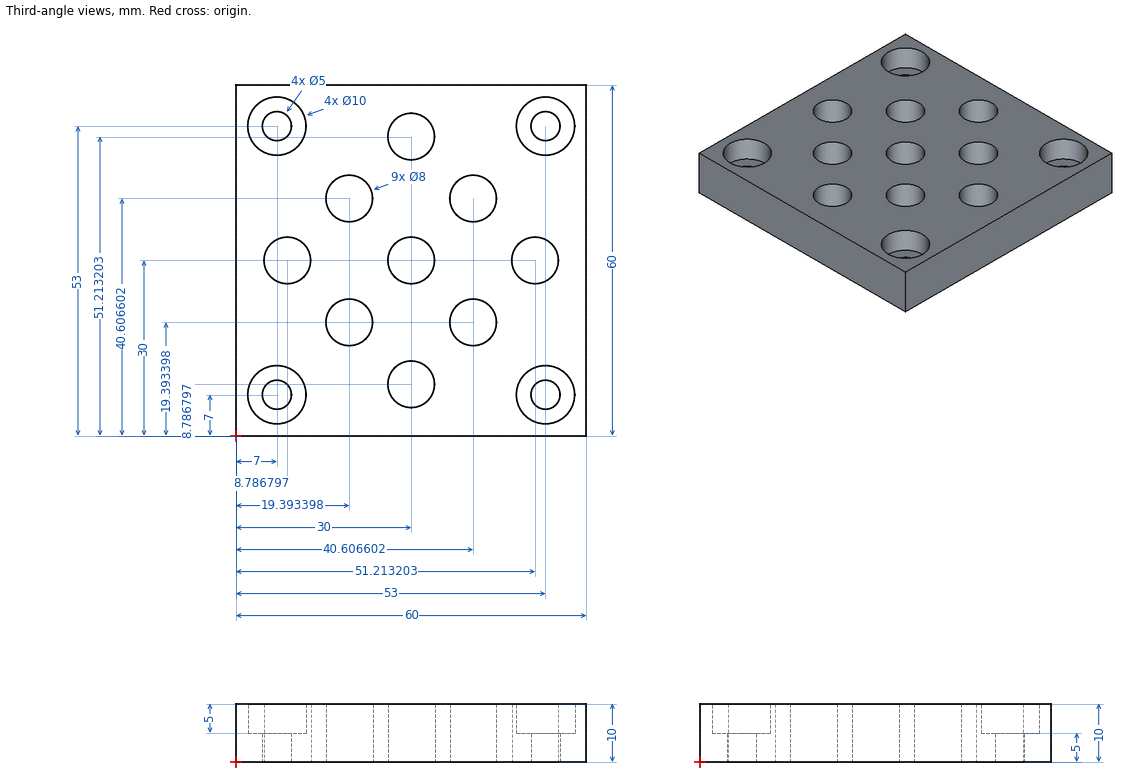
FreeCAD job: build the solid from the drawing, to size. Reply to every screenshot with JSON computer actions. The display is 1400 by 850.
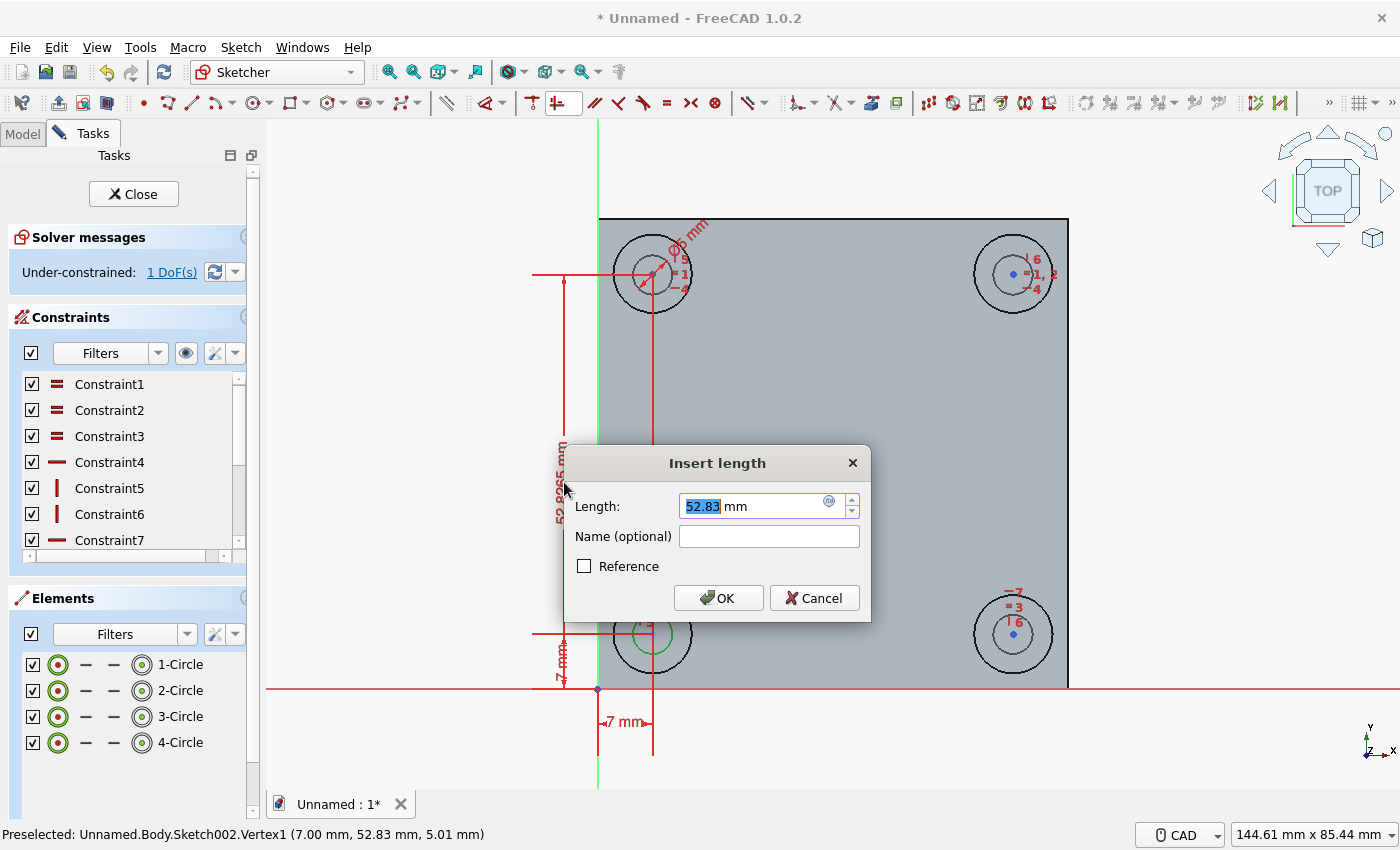
{"action": "type", "text": "53"}
{"action": "key", "text": "Return"}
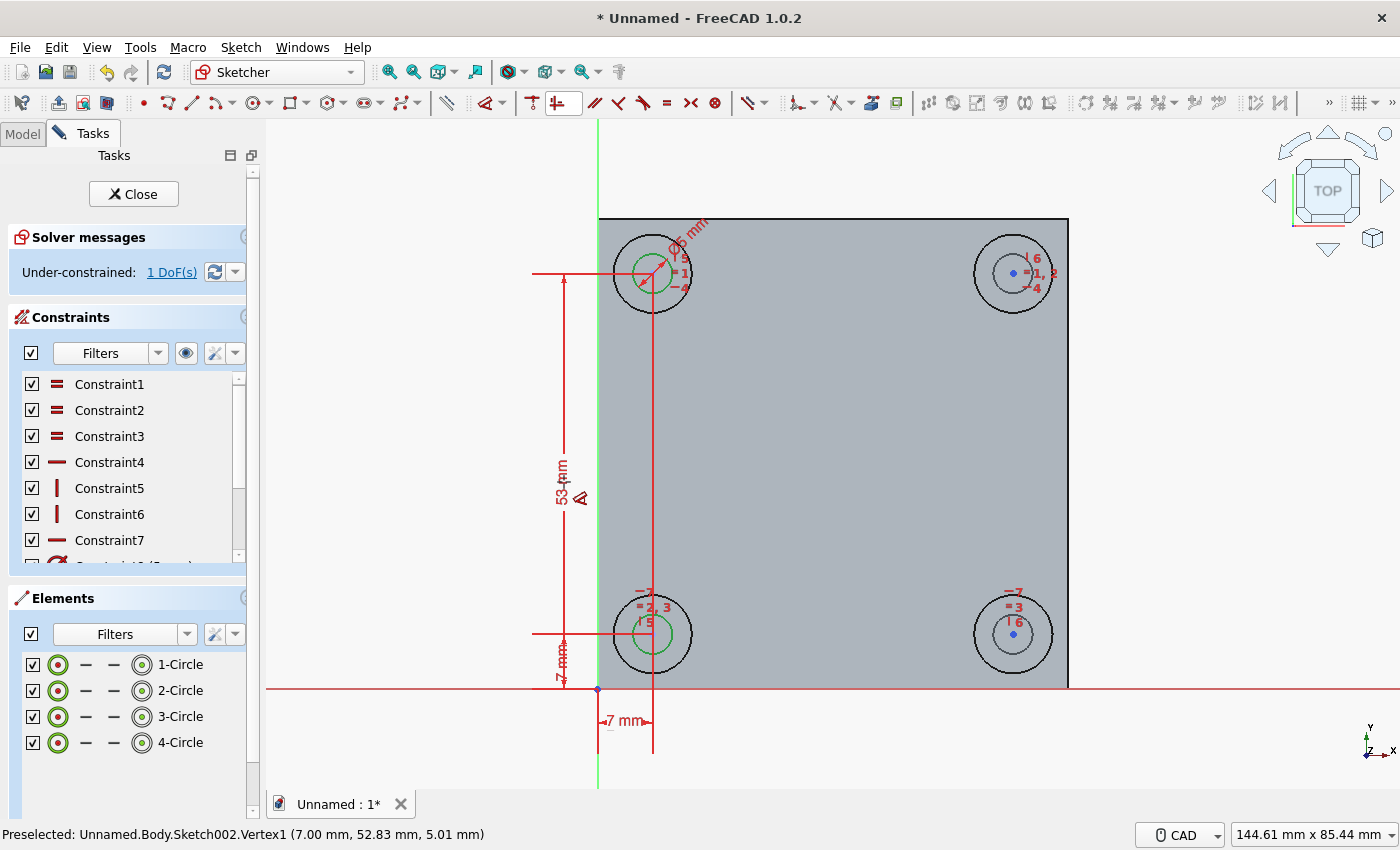
{"action": "left_click", "coordinate": [1013, 274]}
{"action": "left_click", "coordinate": [805, 723]}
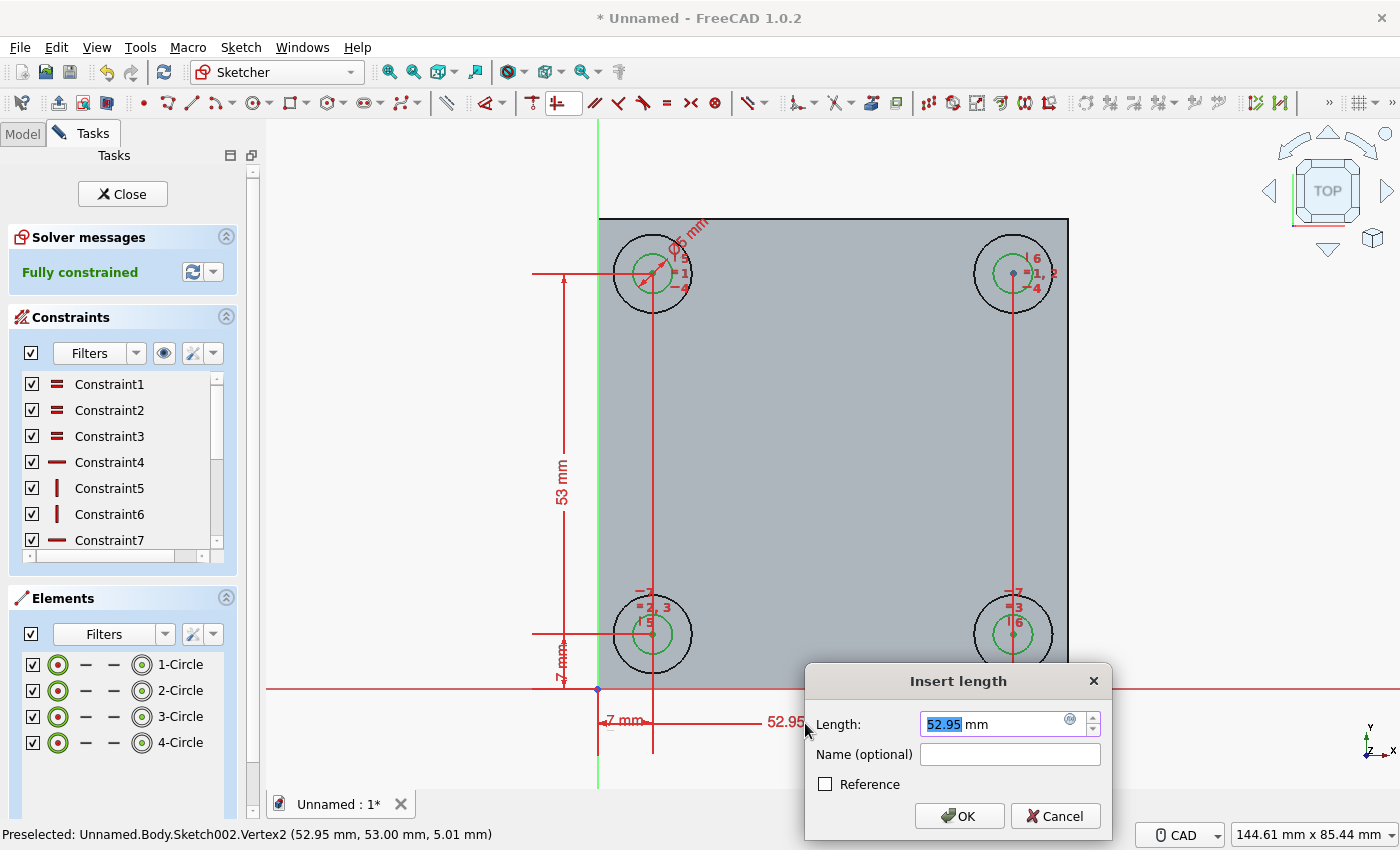
{"action": "type", "text": "53"}
{"action": "key", "text": "Return"}
{"action": "key", "text": "Escape"}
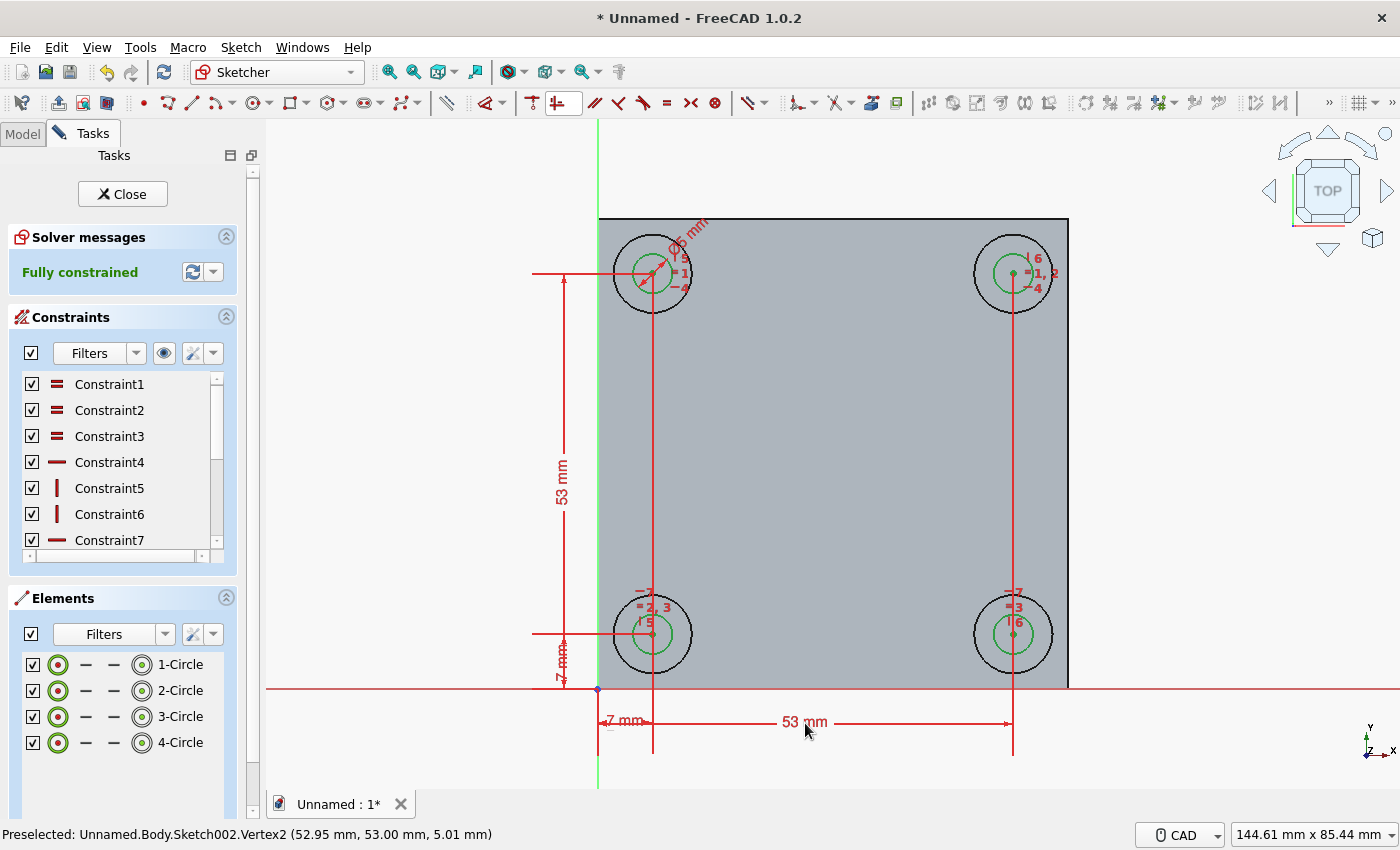
{"action": "left_click", "coordinate": [123, 194]}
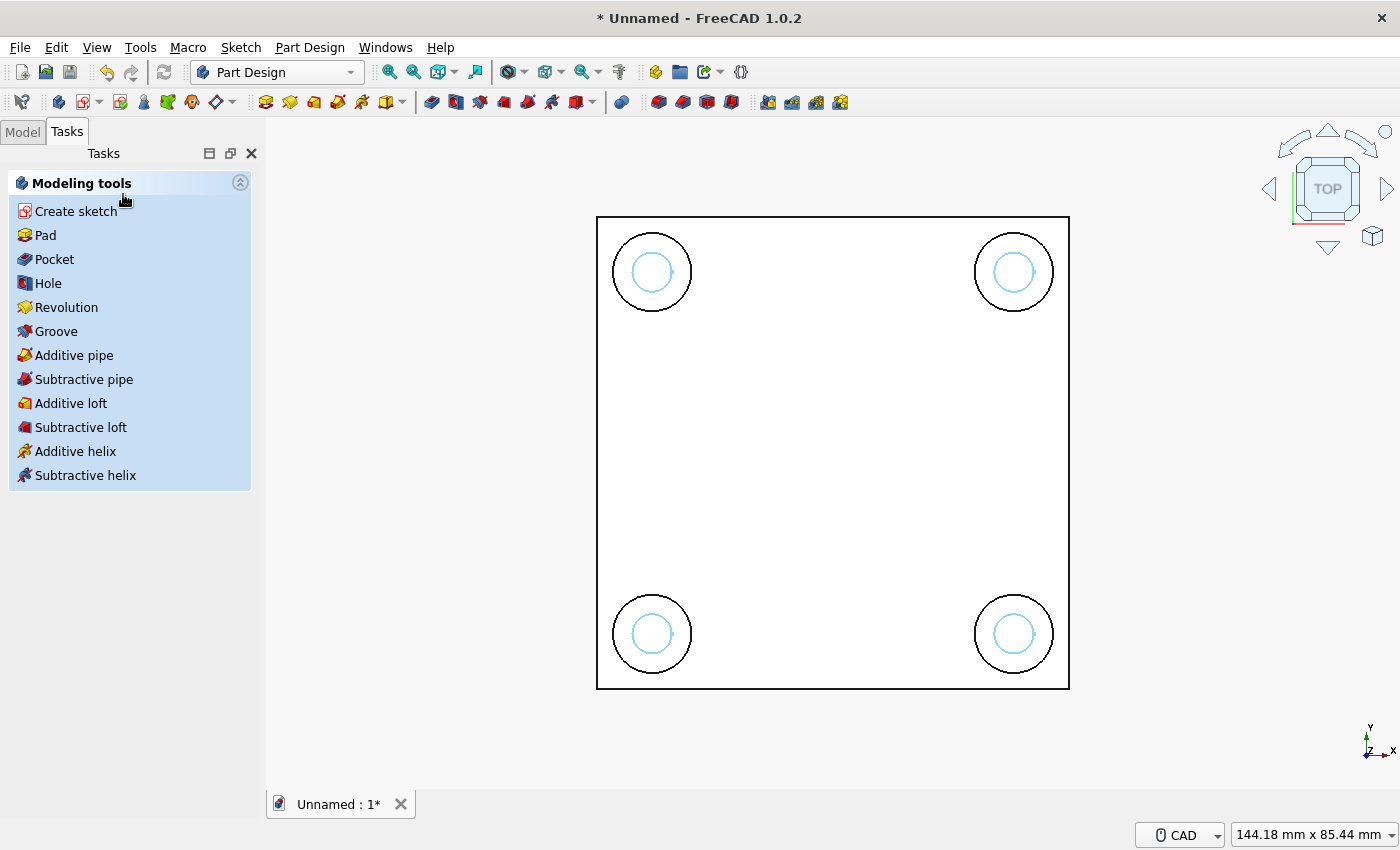
{"action": "left_click", "coordinate": [432, 102]}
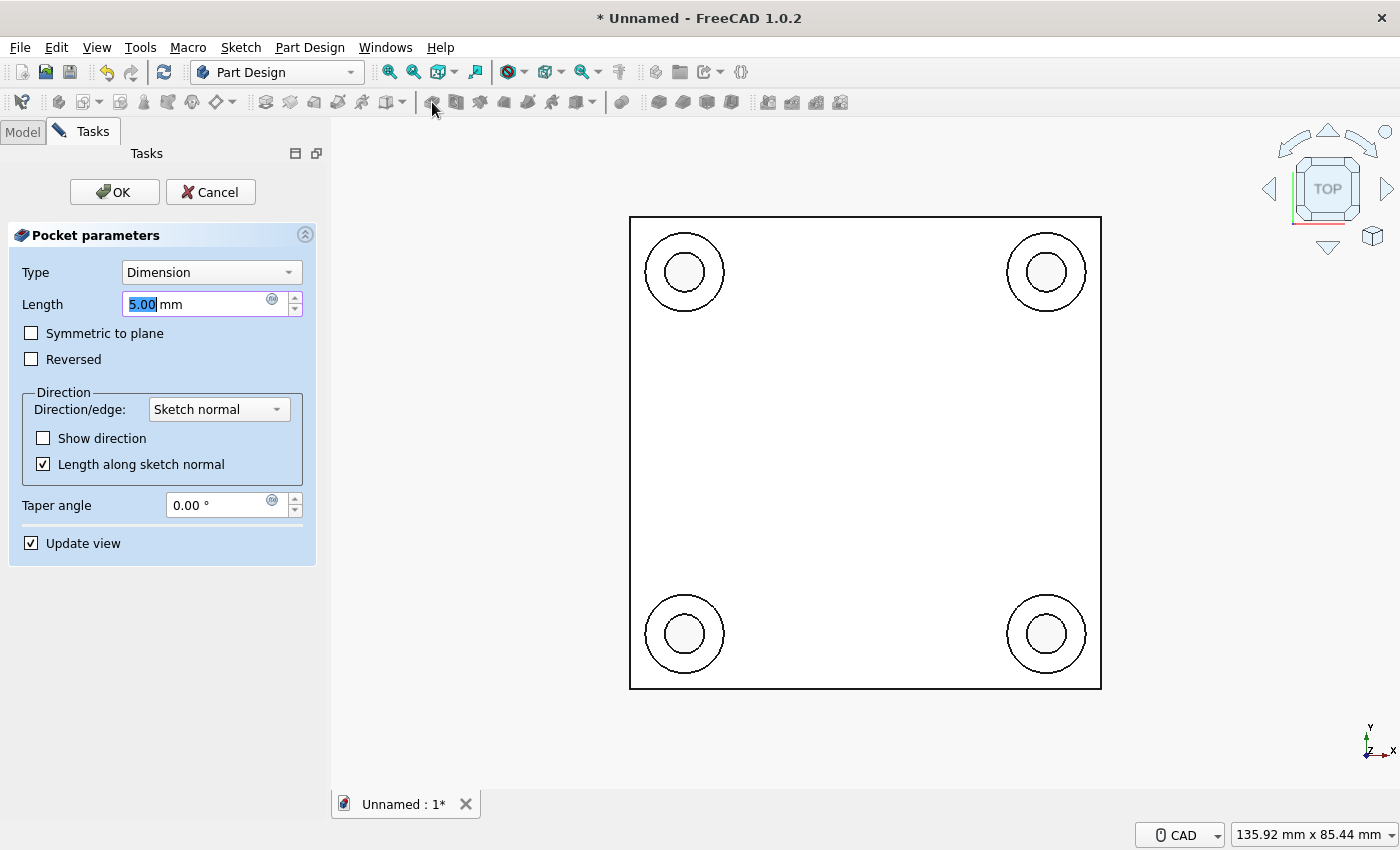
{"action": "type", "text": "5"}
{"action": "key", "text": "Tab"}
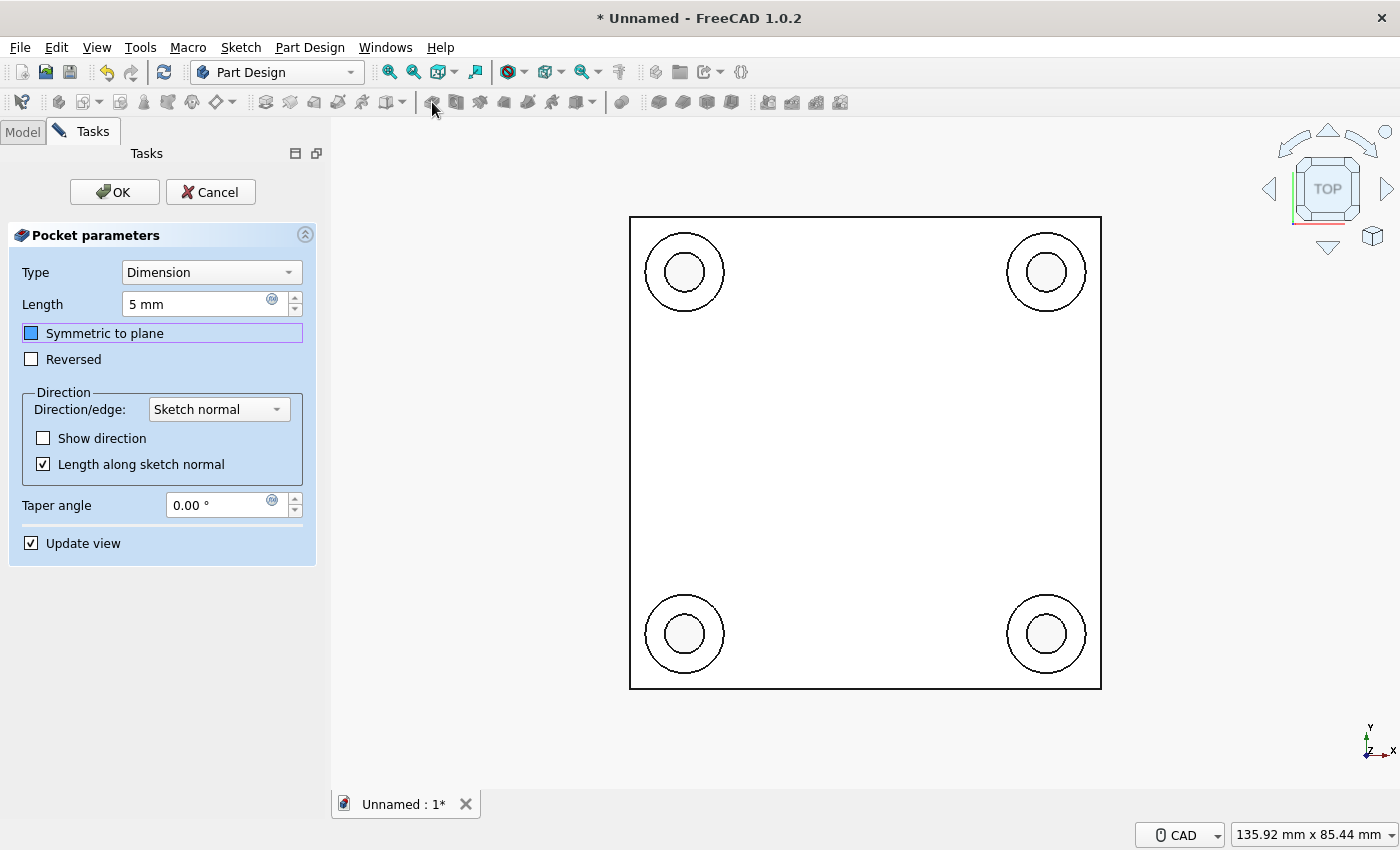
{"action": "left_click", "coordinate": [115, 192]}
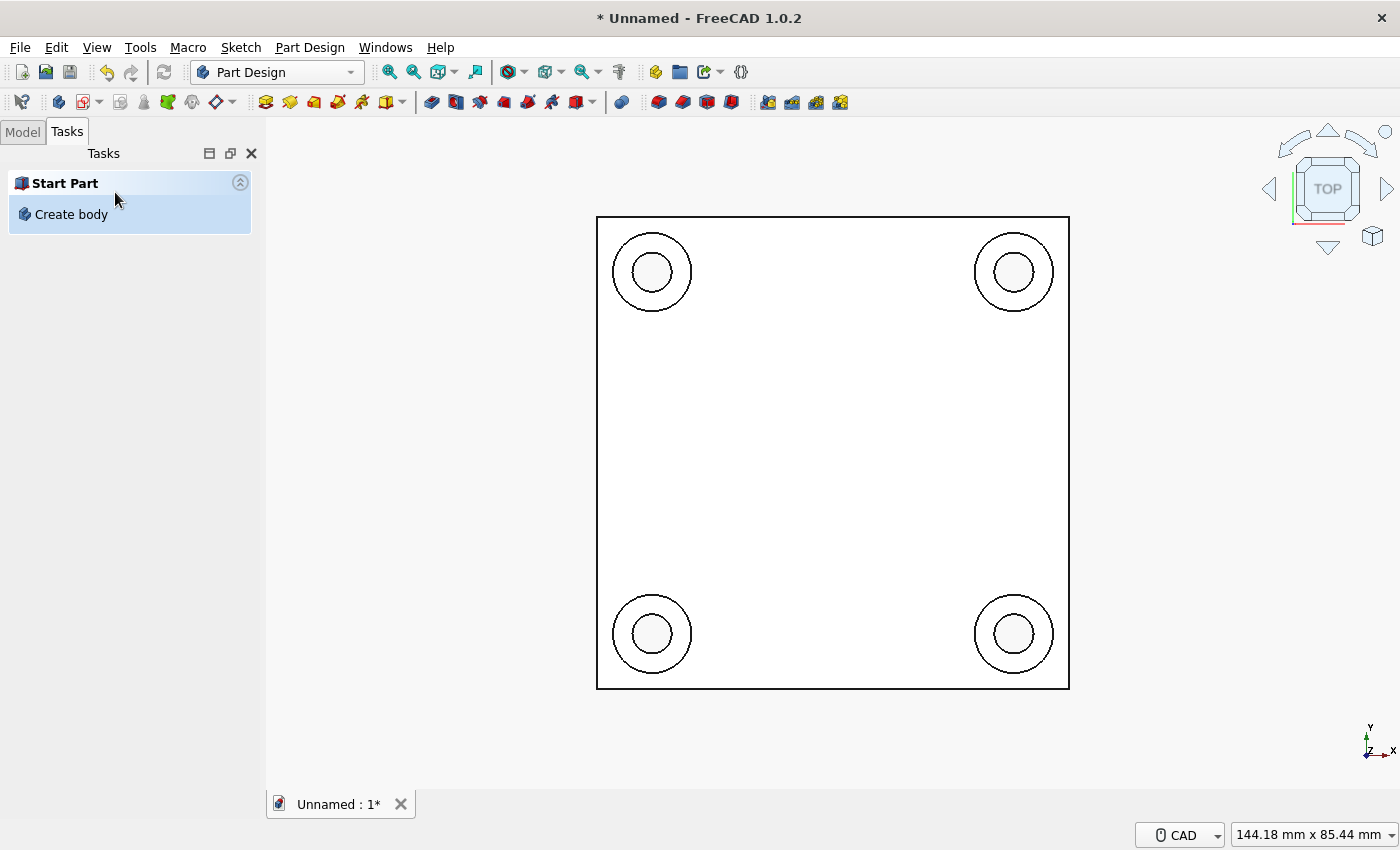
{"action": "left_click", "coordinate": [833, 452]}